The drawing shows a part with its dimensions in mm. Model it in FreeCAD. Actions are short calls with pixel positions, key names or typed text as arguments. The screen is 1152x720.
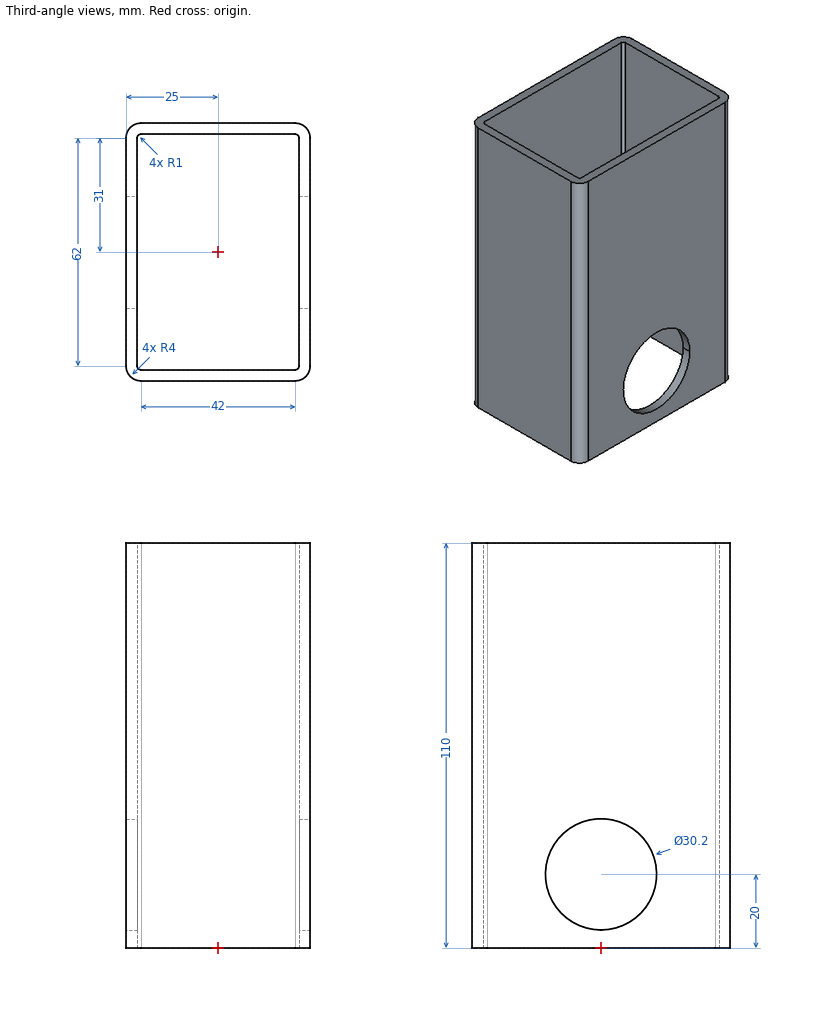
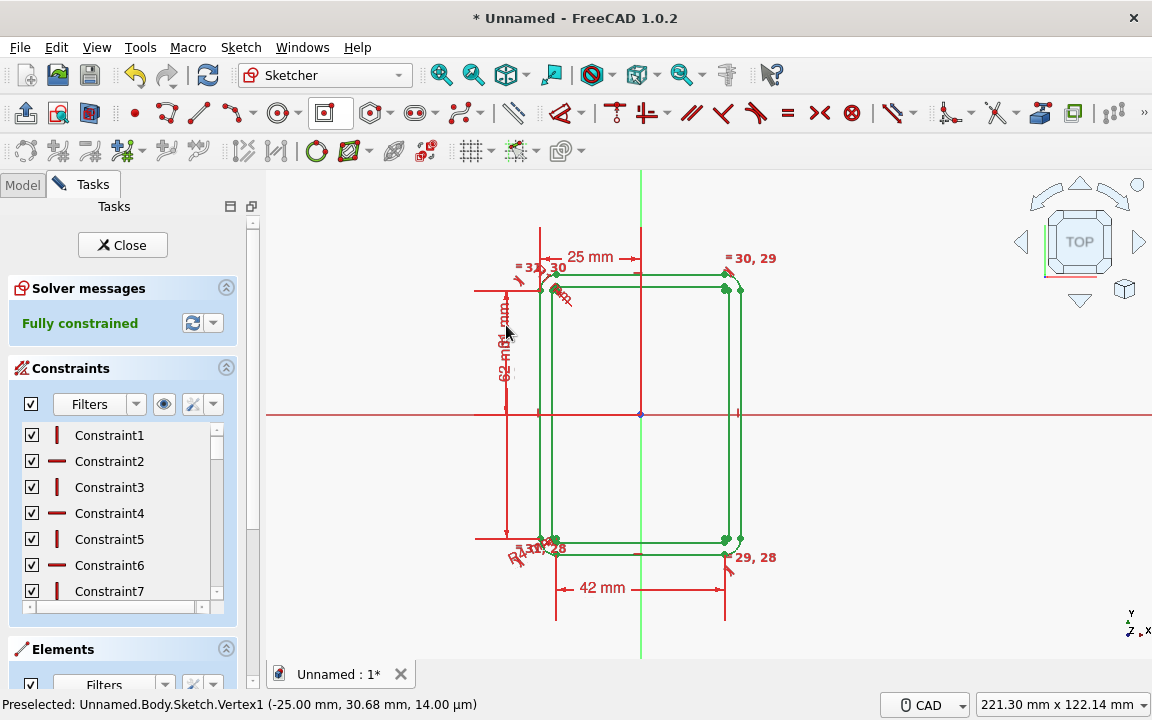
click(123, 245)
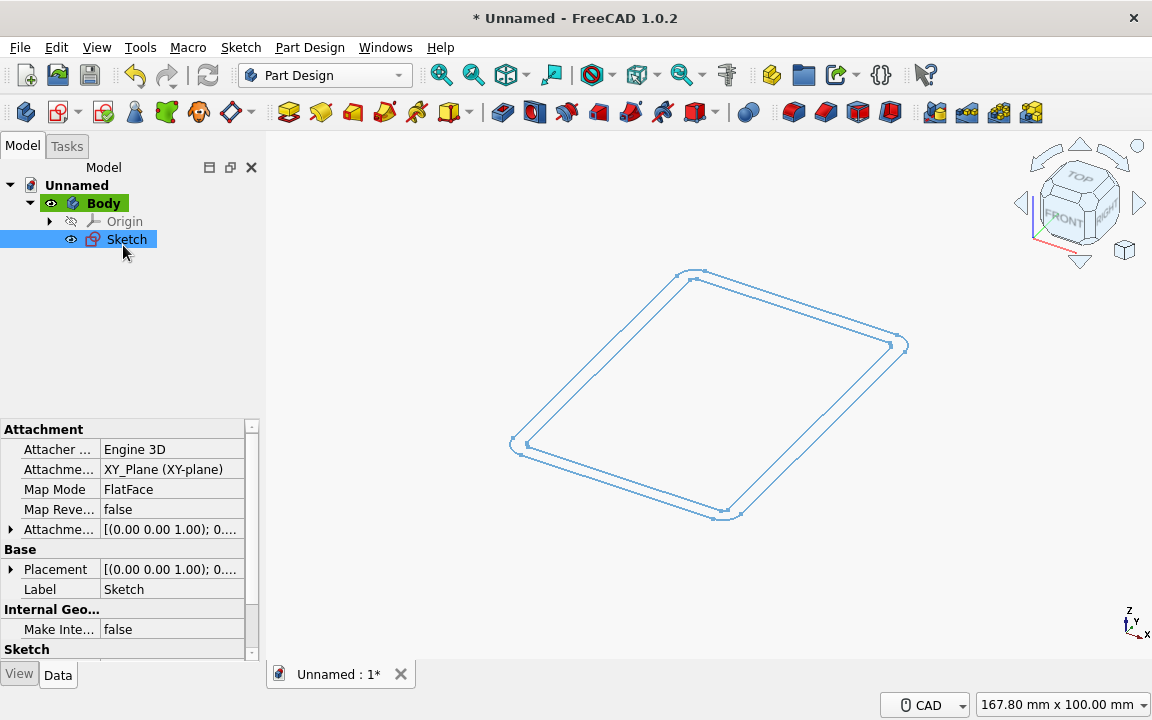
click(290, 112)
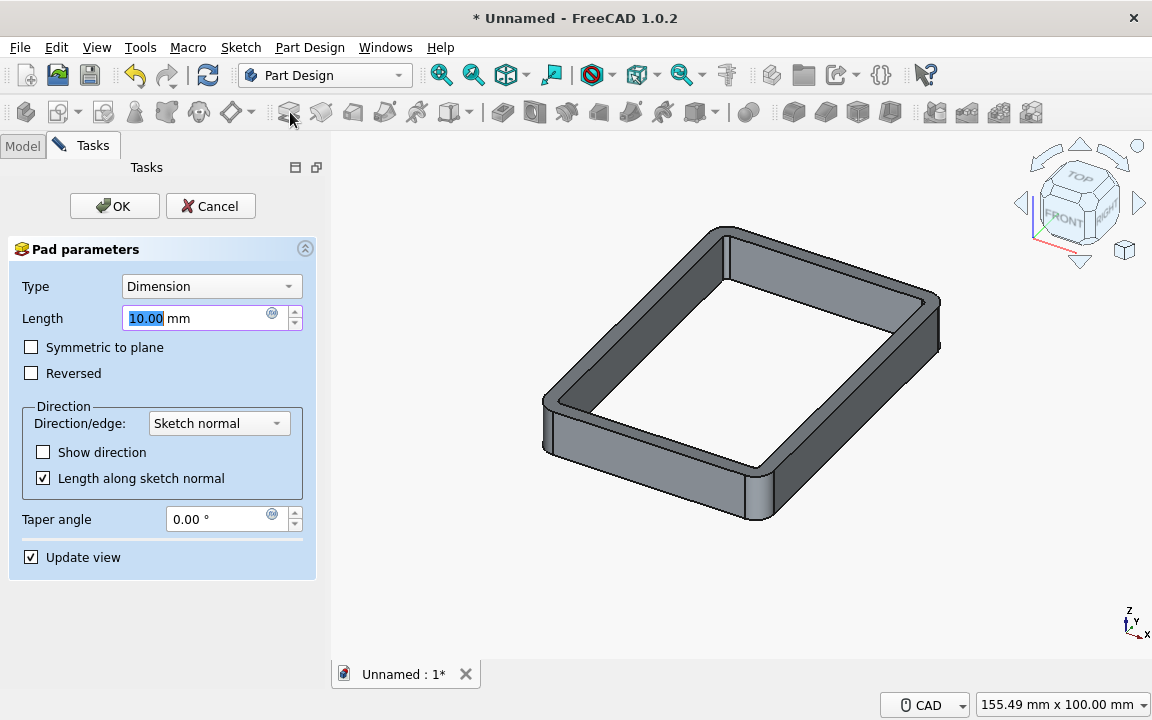
text(110)
key(Tab)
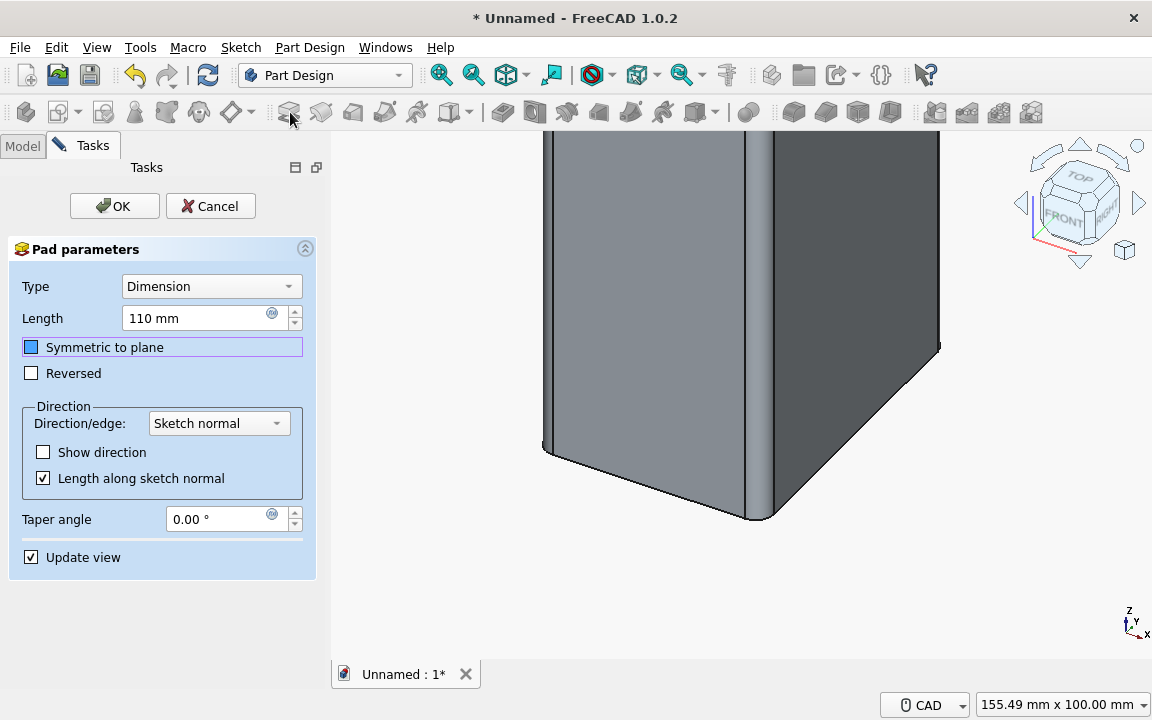
click(115, 206)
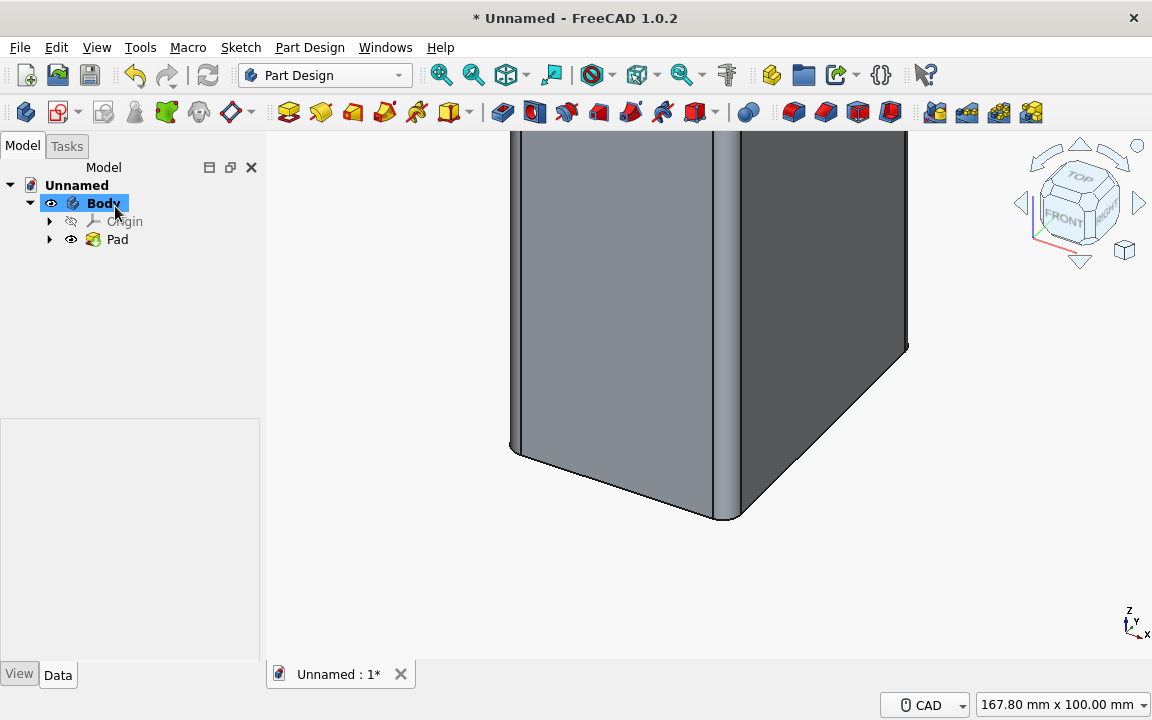
key(v)
key(f)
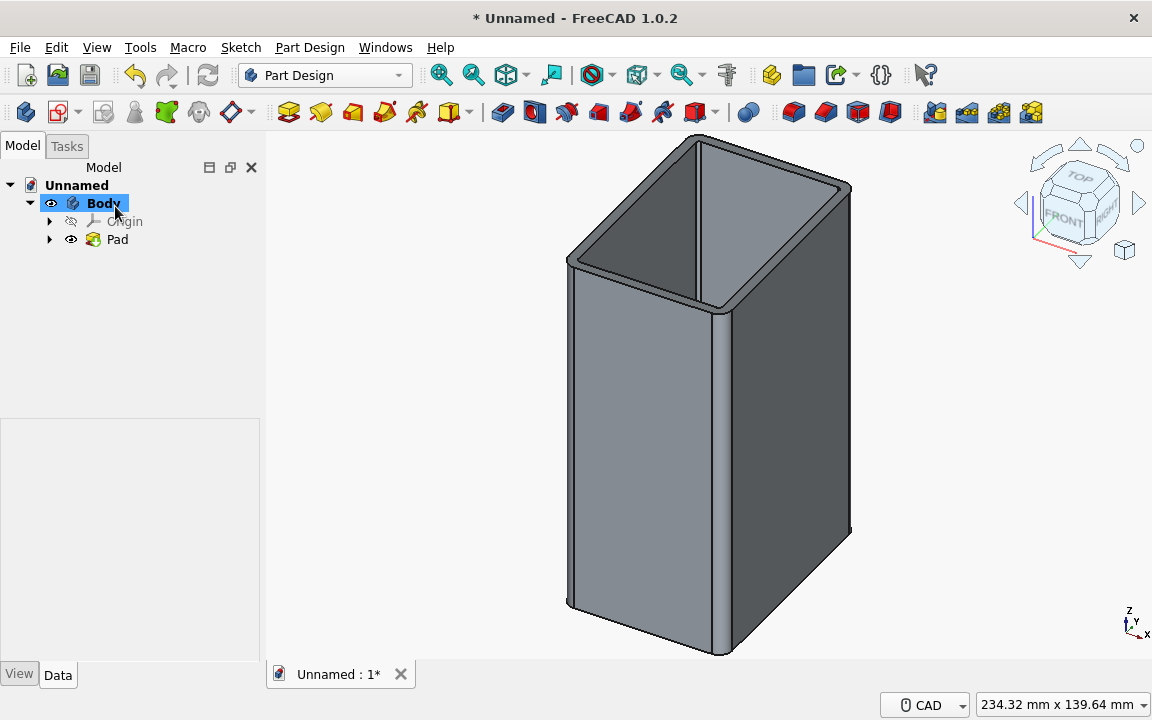
click(791, 372)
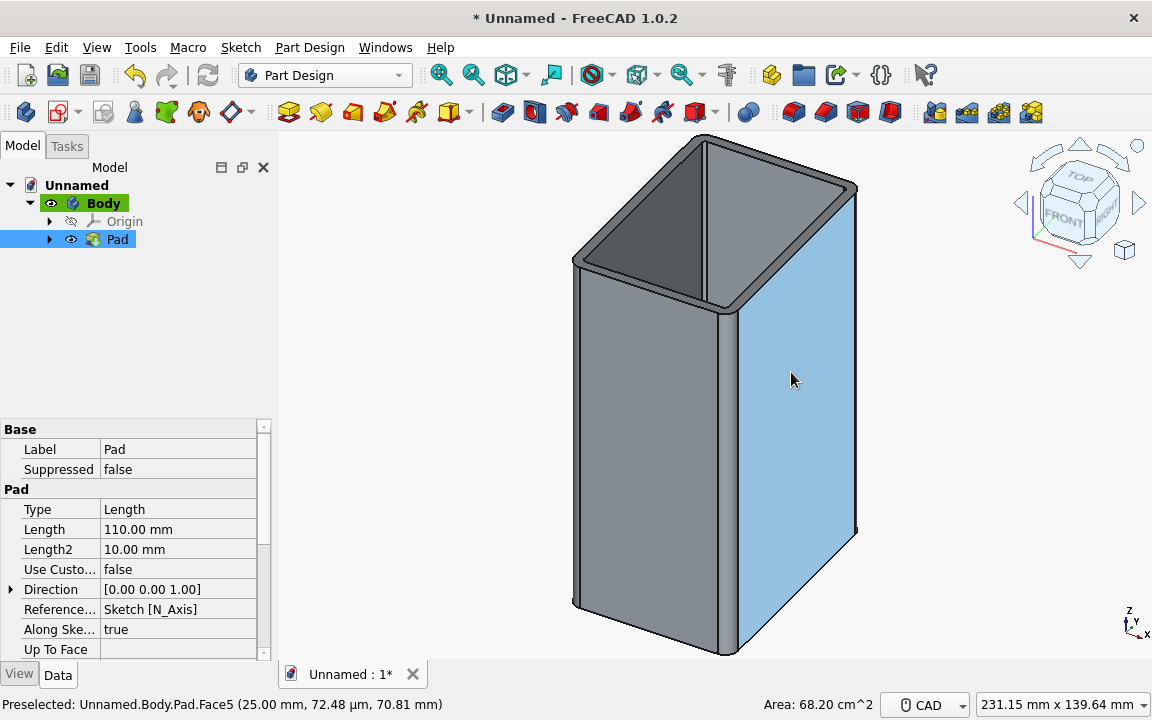
click(58, 112)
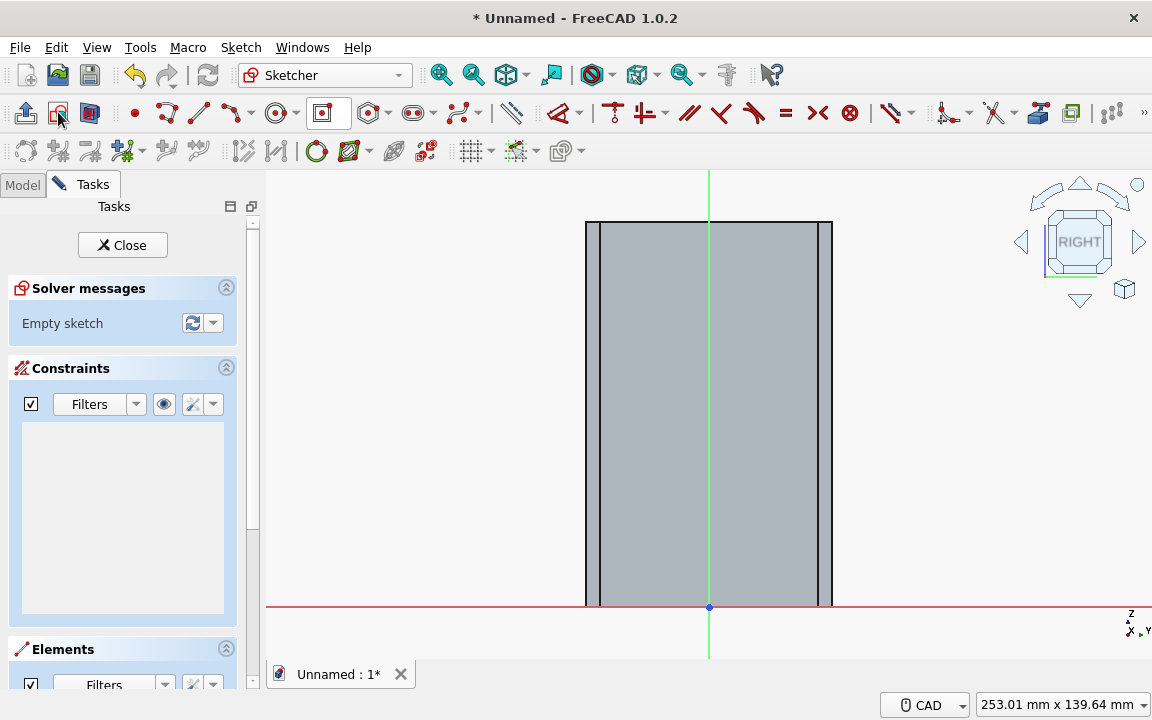
scroll(749, 622, up, 5)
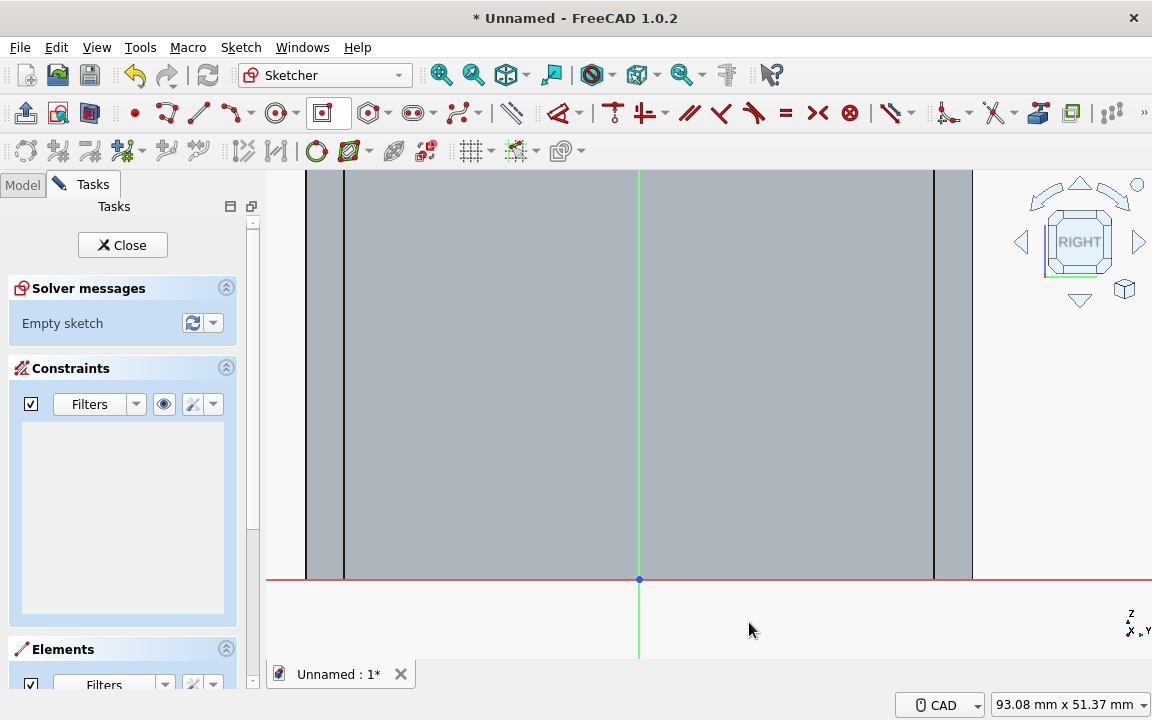
click(276, 114)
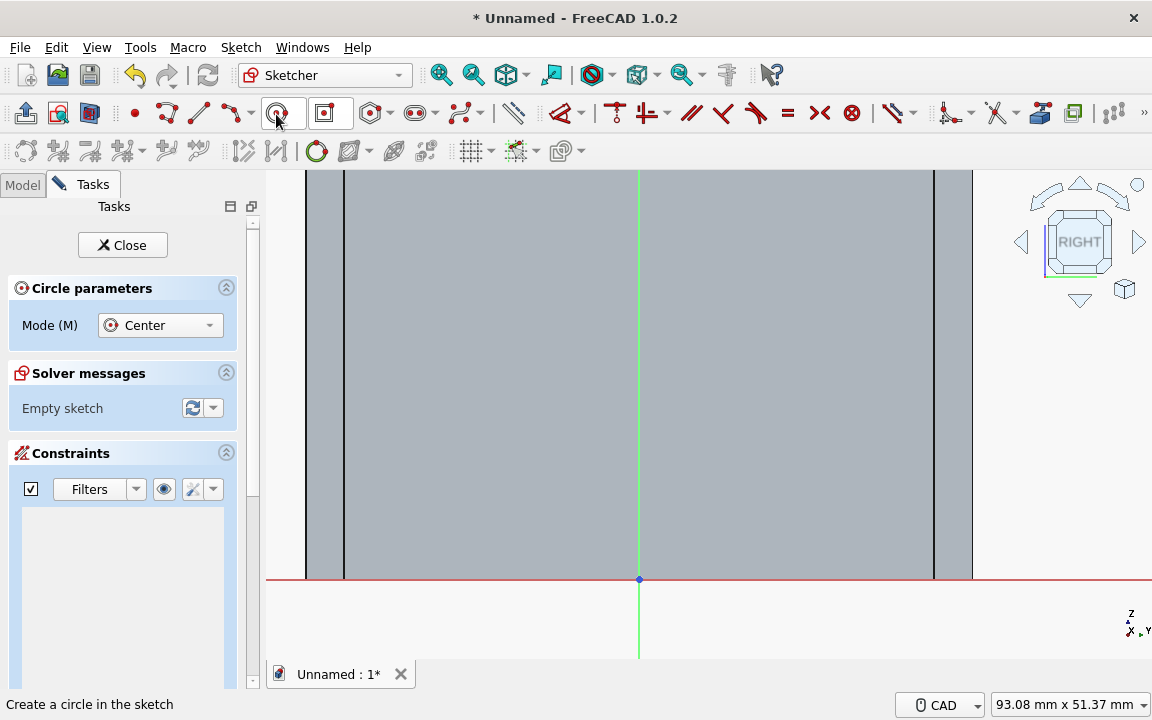
click(639, 390)
move(741, 288)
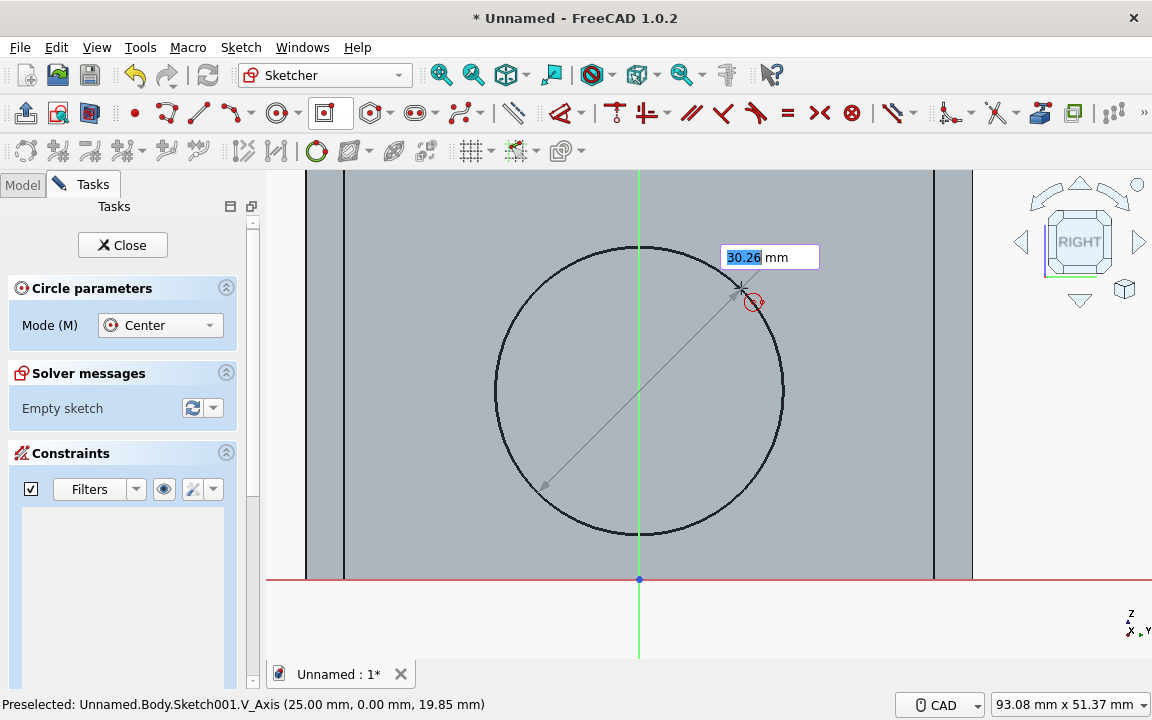
text(30.2)
key(Return)
key(Escape)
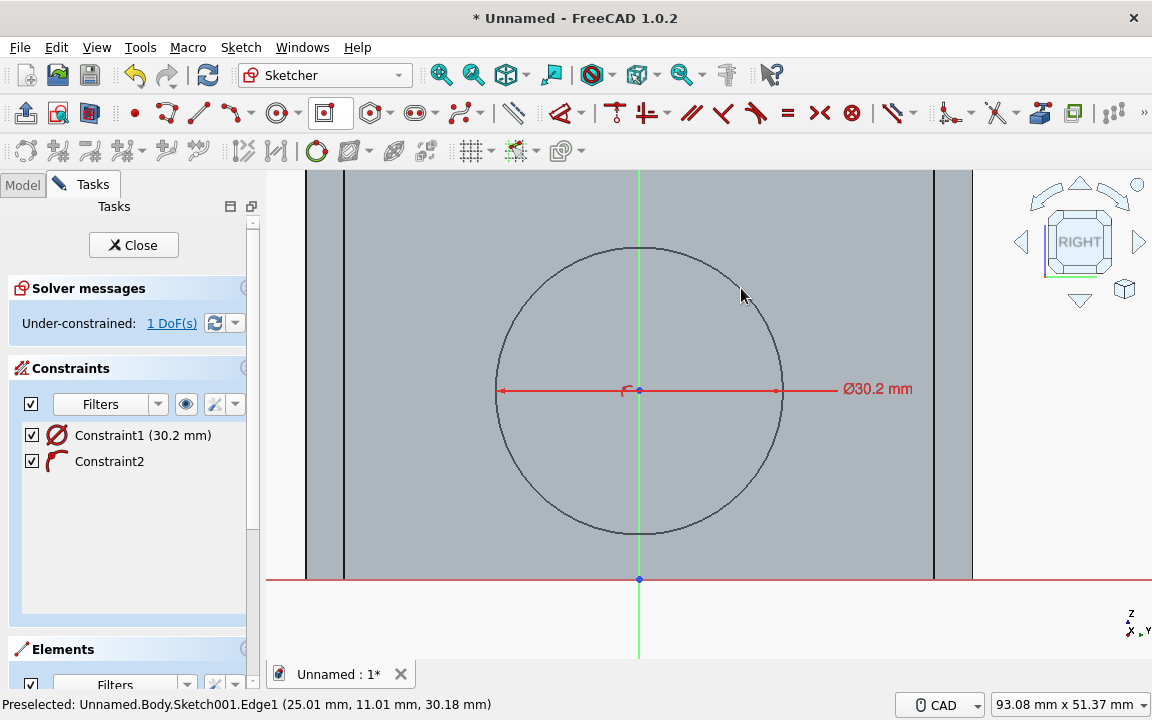
key(d)